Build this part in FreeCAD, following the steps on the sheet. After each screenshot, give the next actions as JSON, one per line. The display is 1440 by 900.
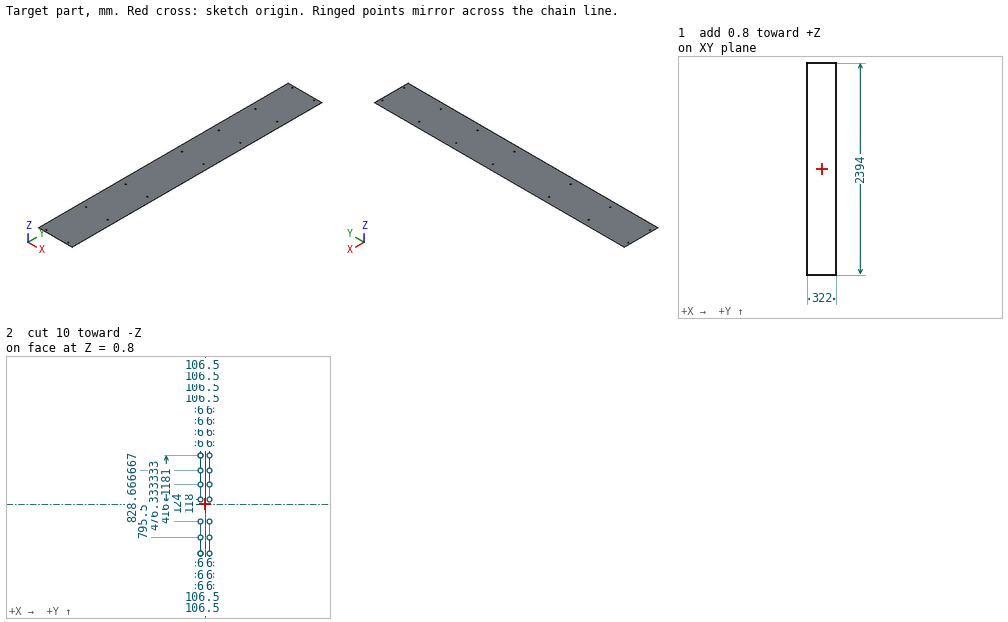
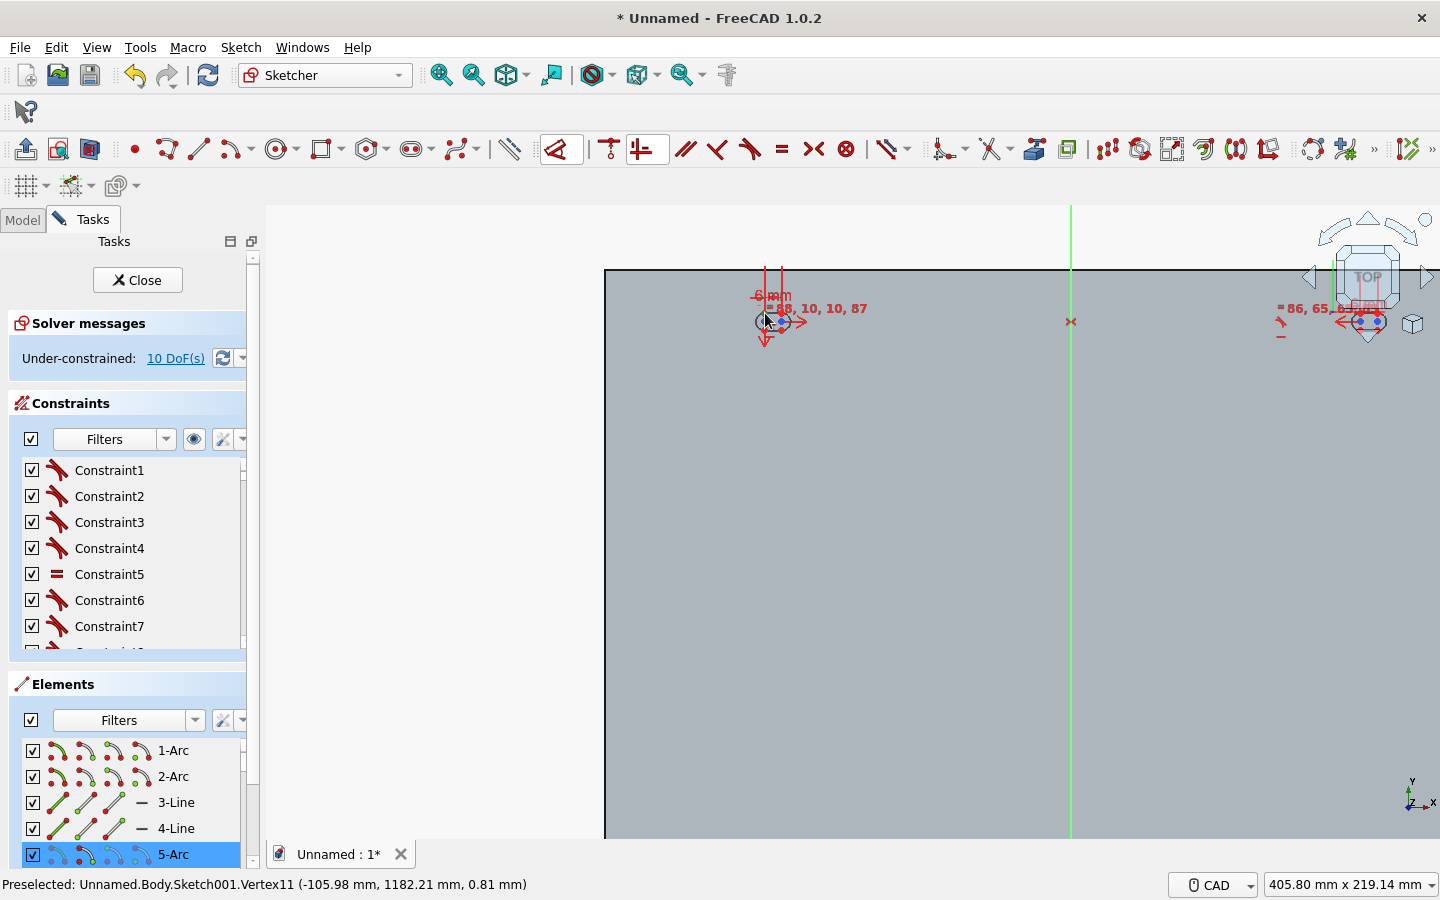
{"action": "key", "text": "i"}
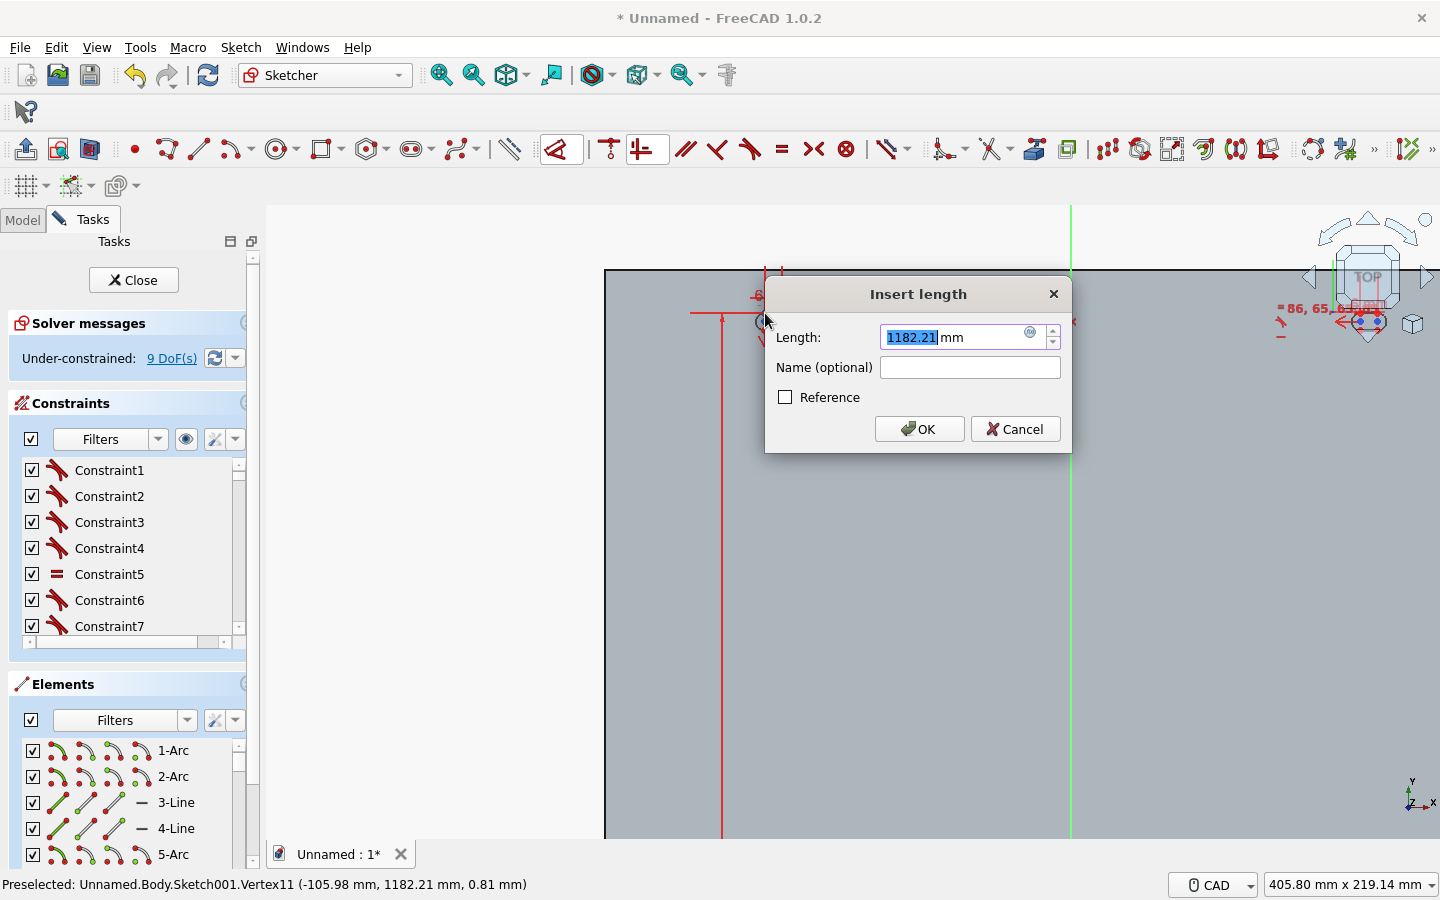
{"action": "type", "text": "1181"}
{"action": "key", "text": "Return"}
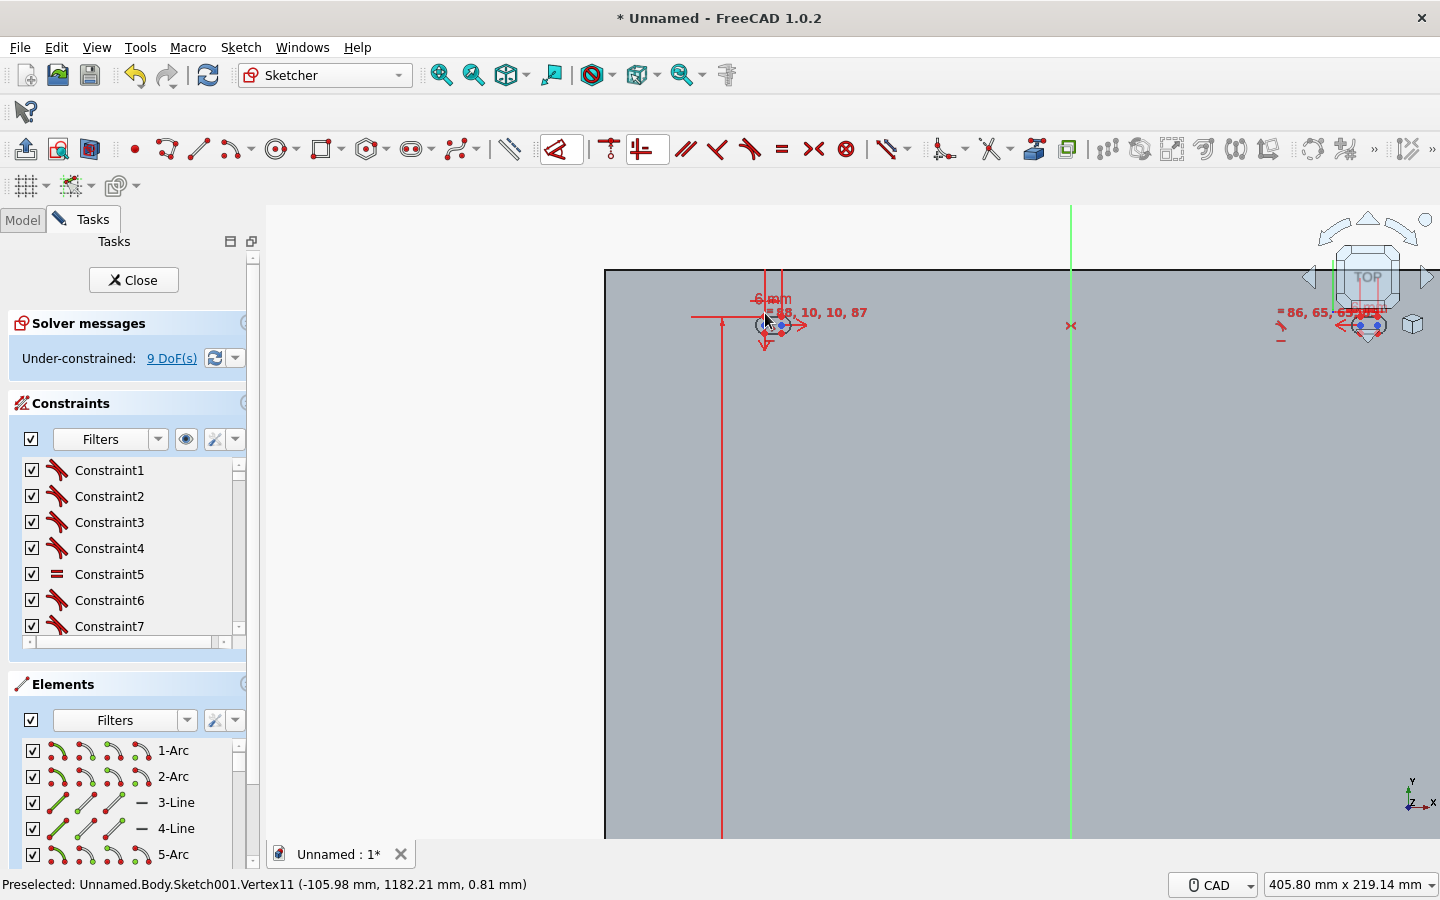
{"action": "scroll", "coordinate": [766, 314], "scroll_direction": "down", "scroll_amount": 14}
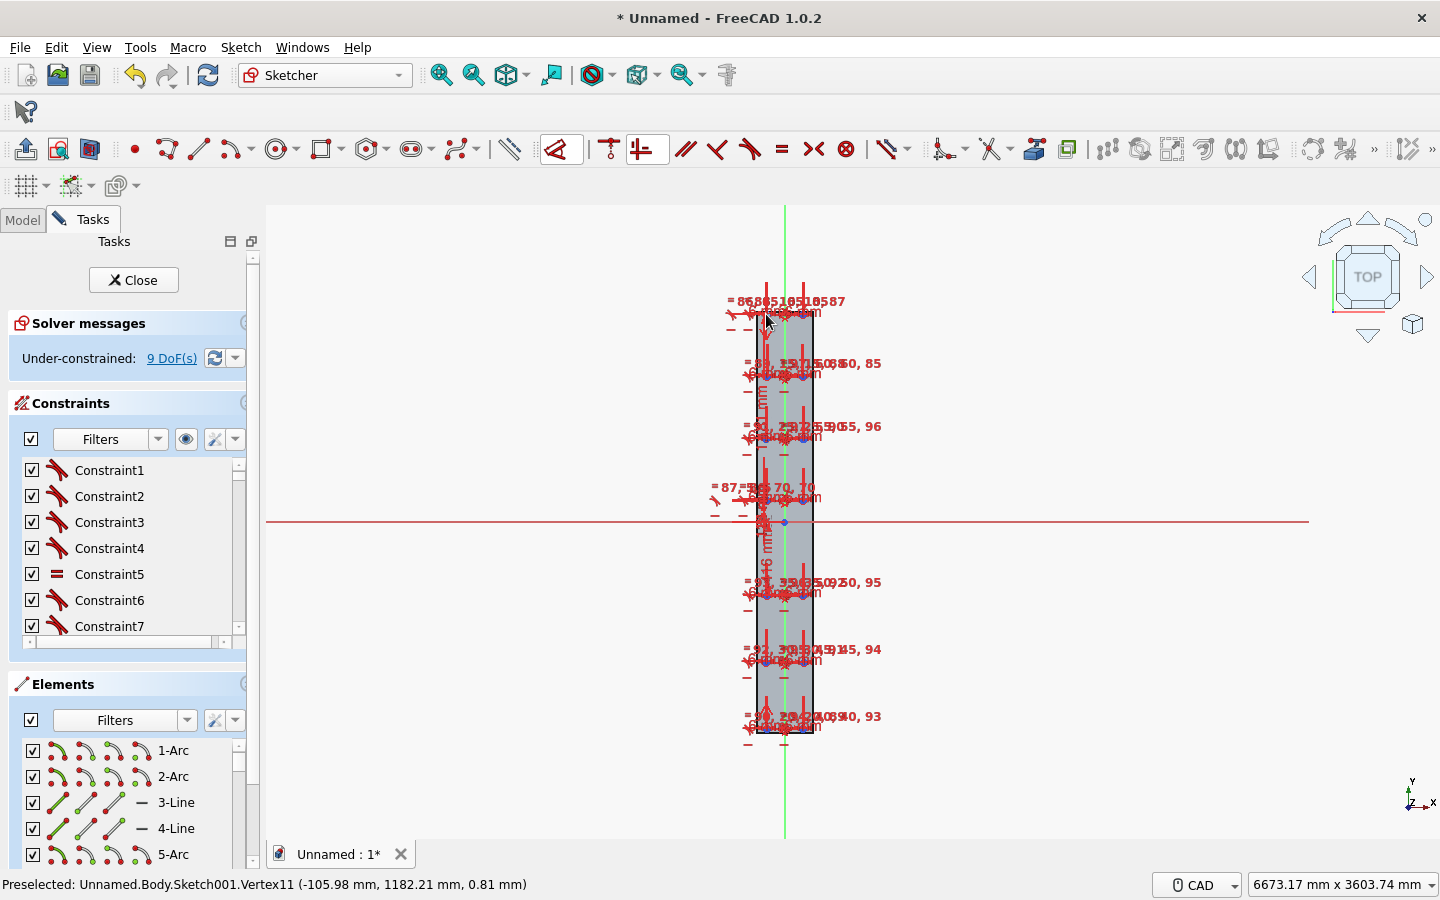
{"action": "scroll", "coordinate": [766, 500], "scroll_direction": "up", "scroll_amount": 14}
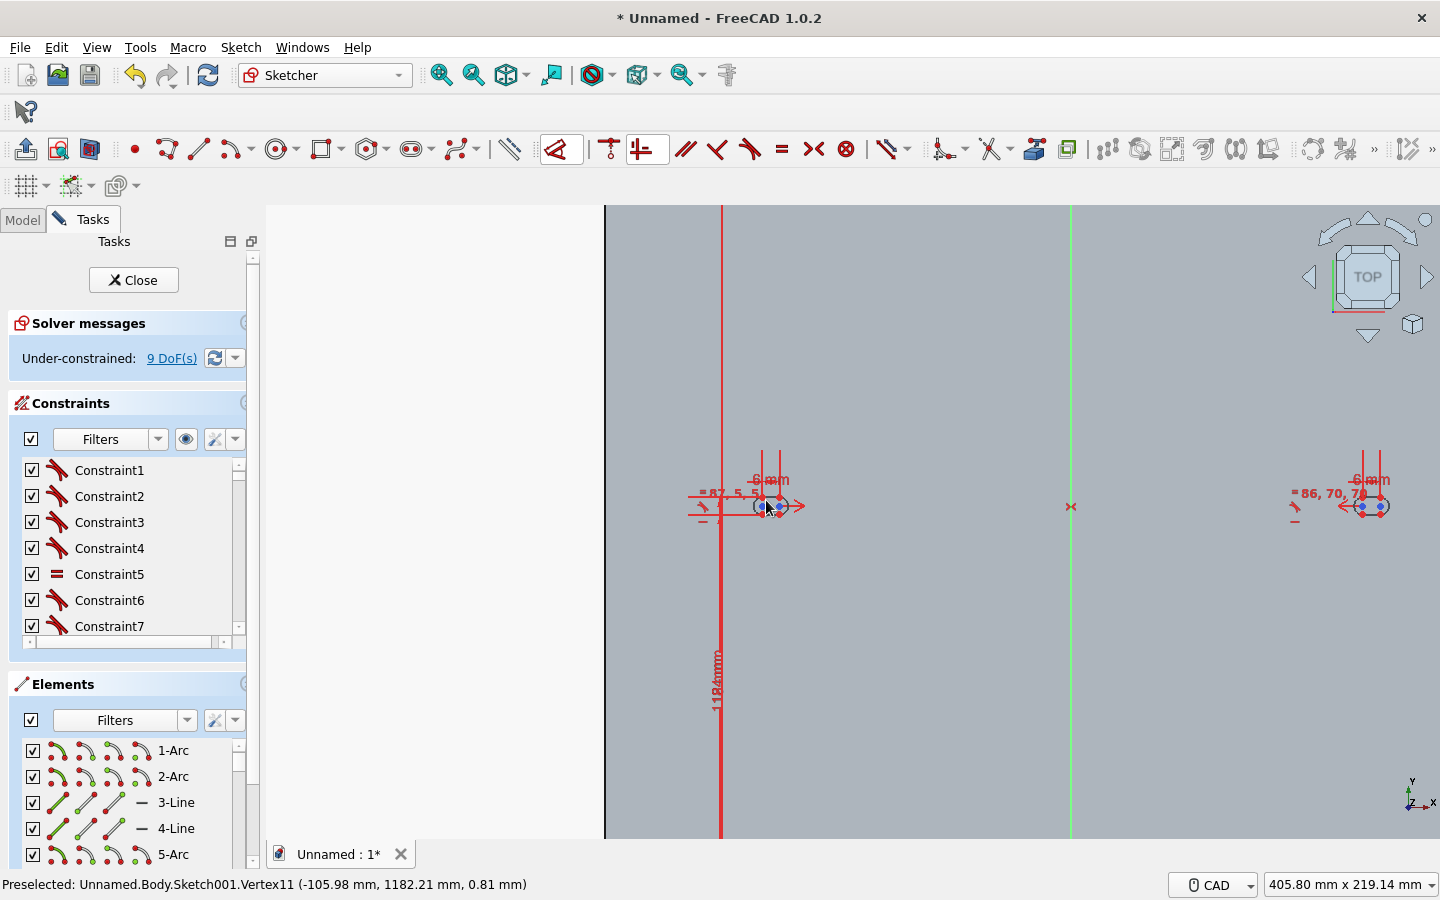
{"action": "left_click", "coordinate": [762, 497]}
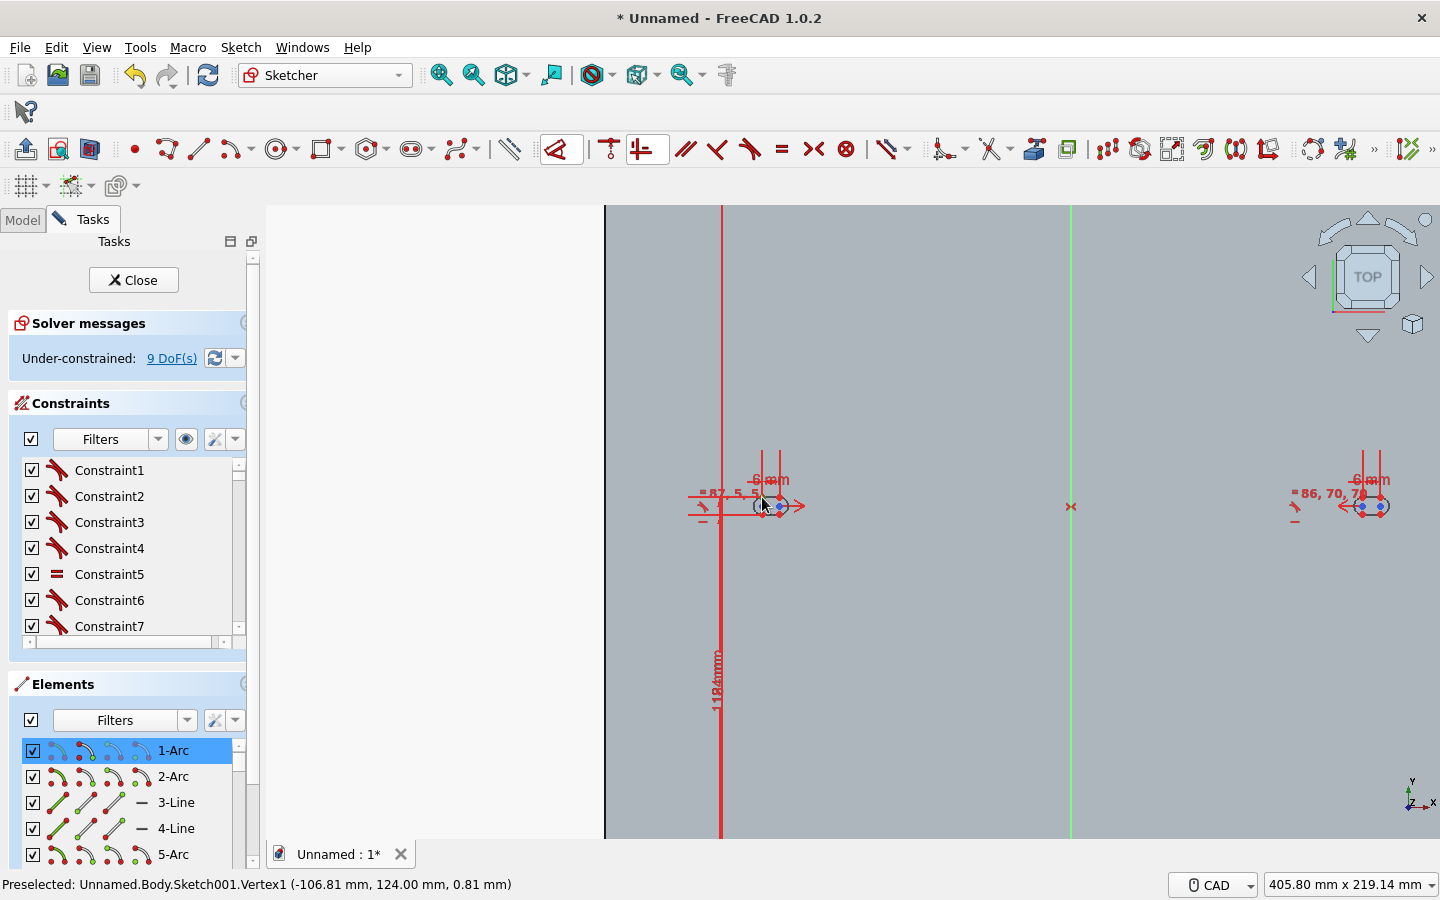
{"action": "key", "text": "l"}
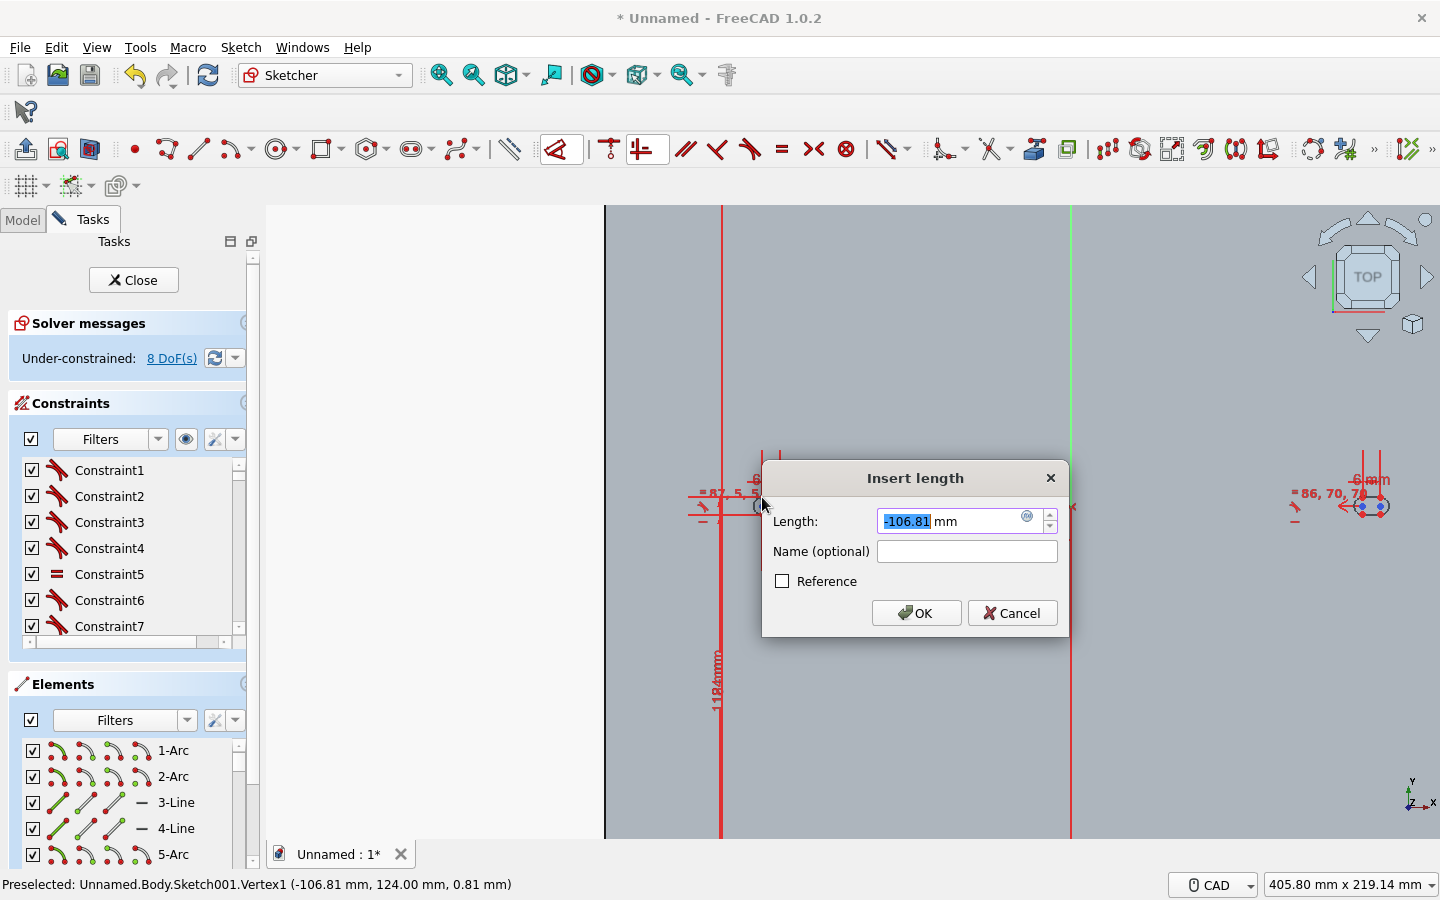
{"action": "type", "text": "-106.5"}
{"action": "key", "text": "Return"}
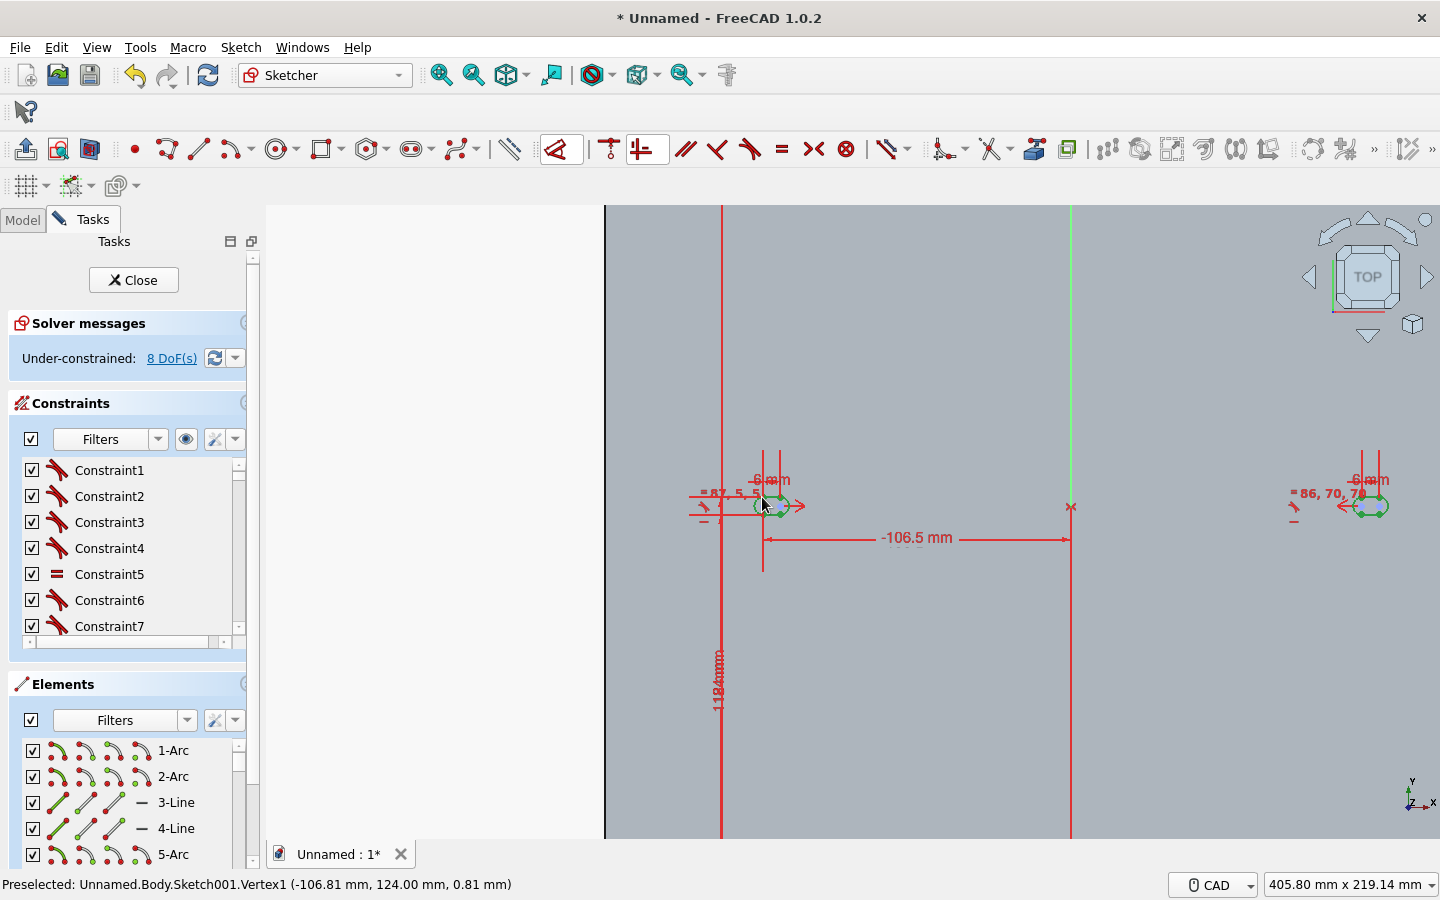
{"action": "scroll", "coordinate": [766, 500], "scroll_direction": "down", "scroll_amount": 14}